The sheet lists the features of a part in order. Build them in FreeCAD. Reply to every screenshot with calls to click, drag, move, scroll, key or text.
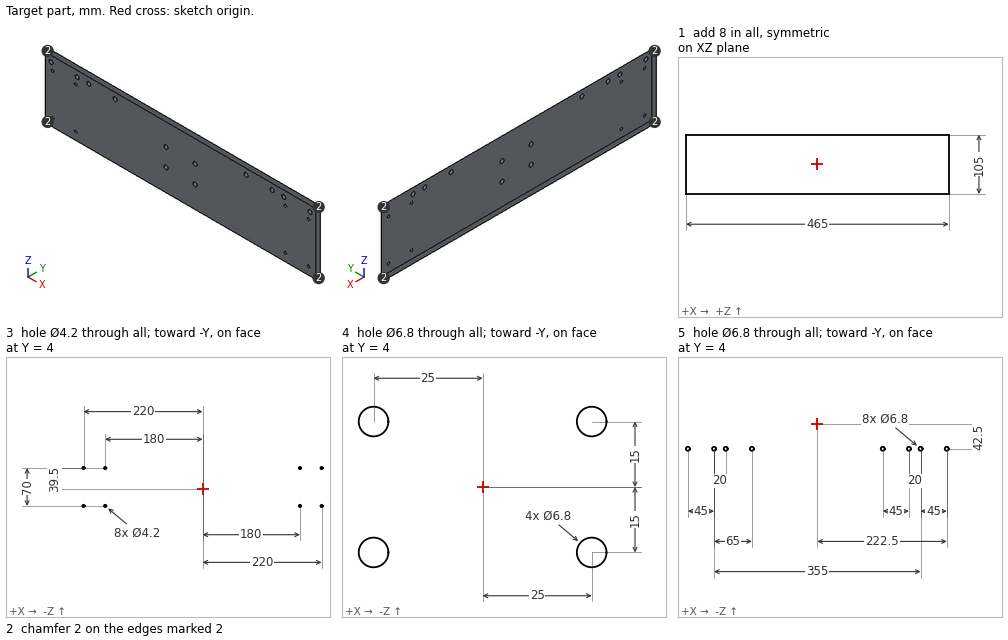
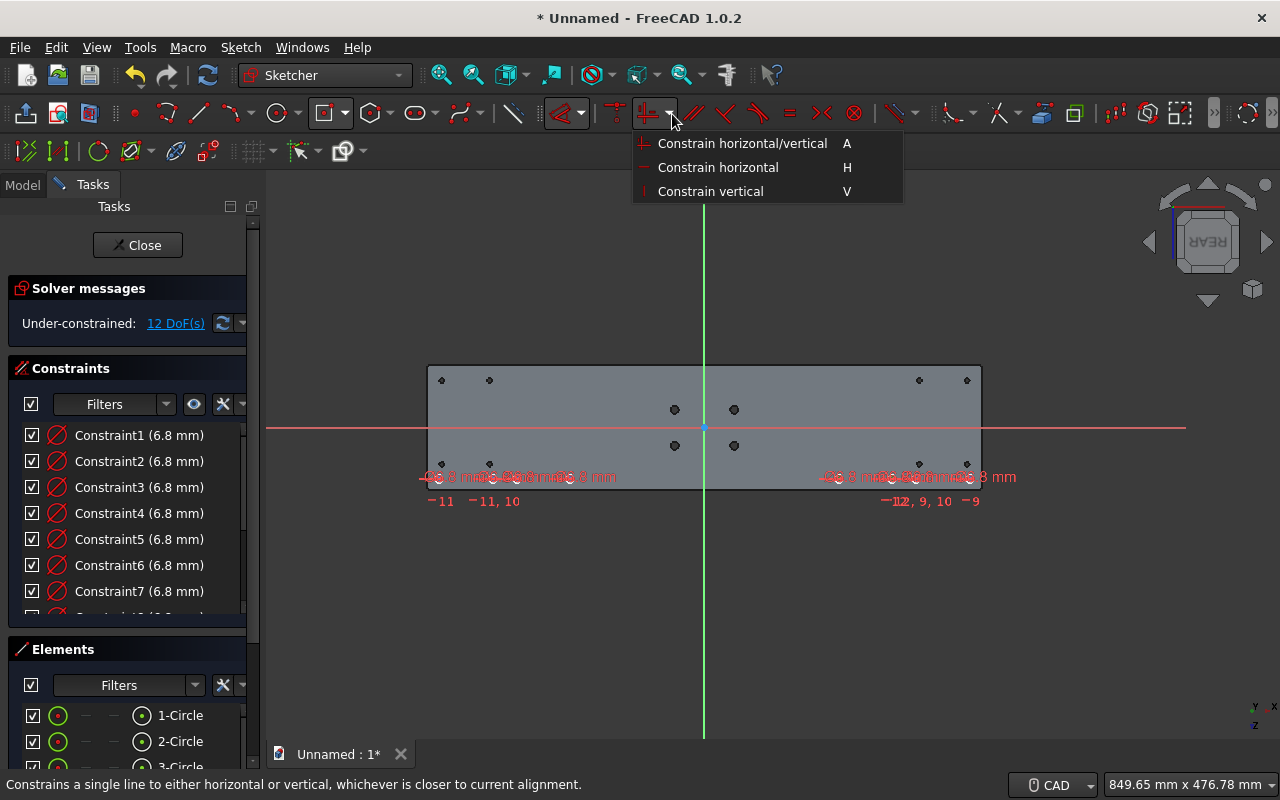
click(768, 167)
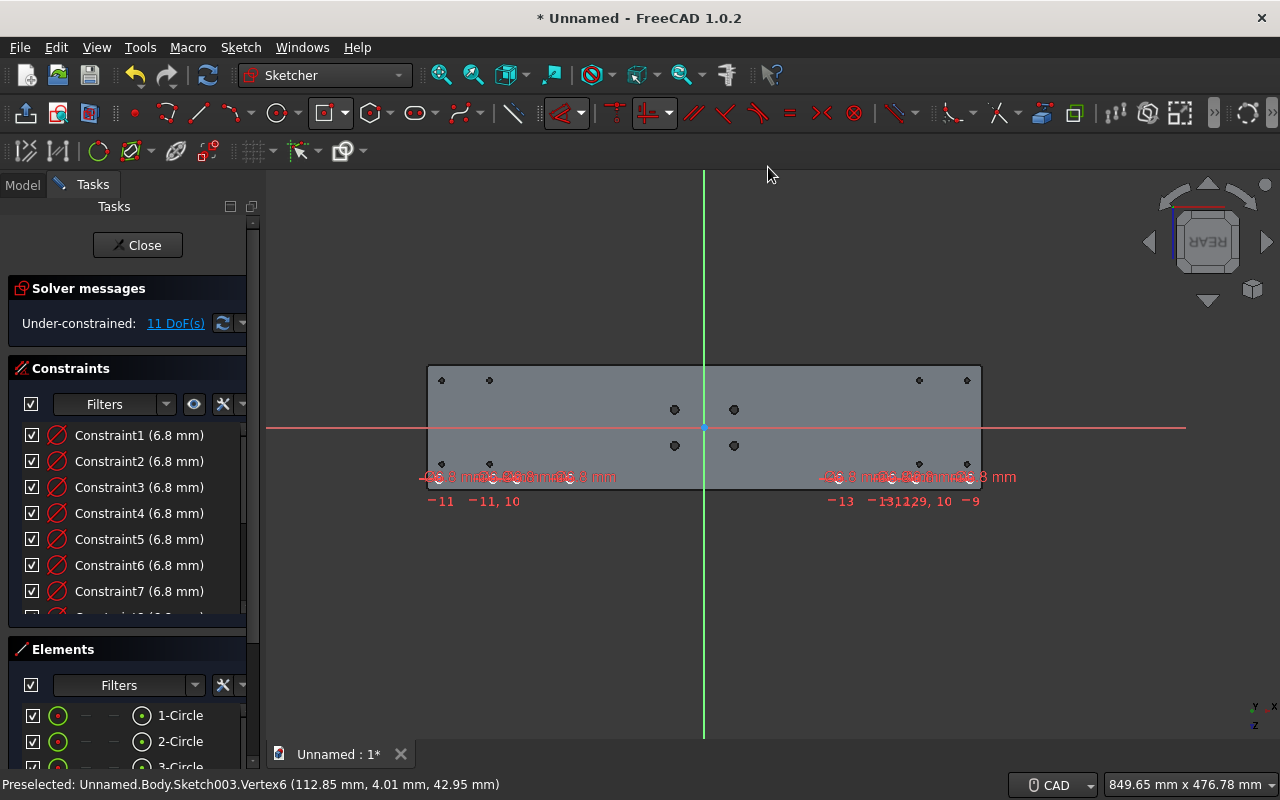
click(493, 479)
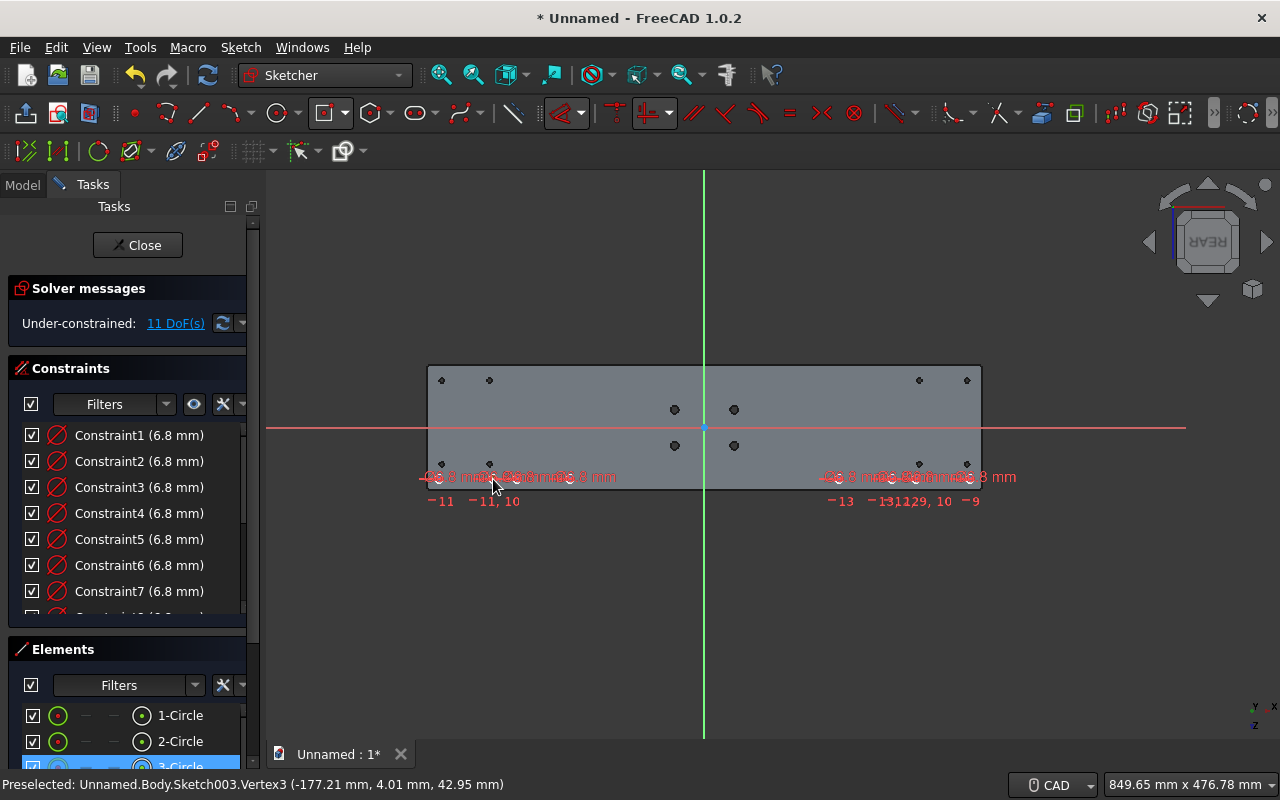
click(570, 479)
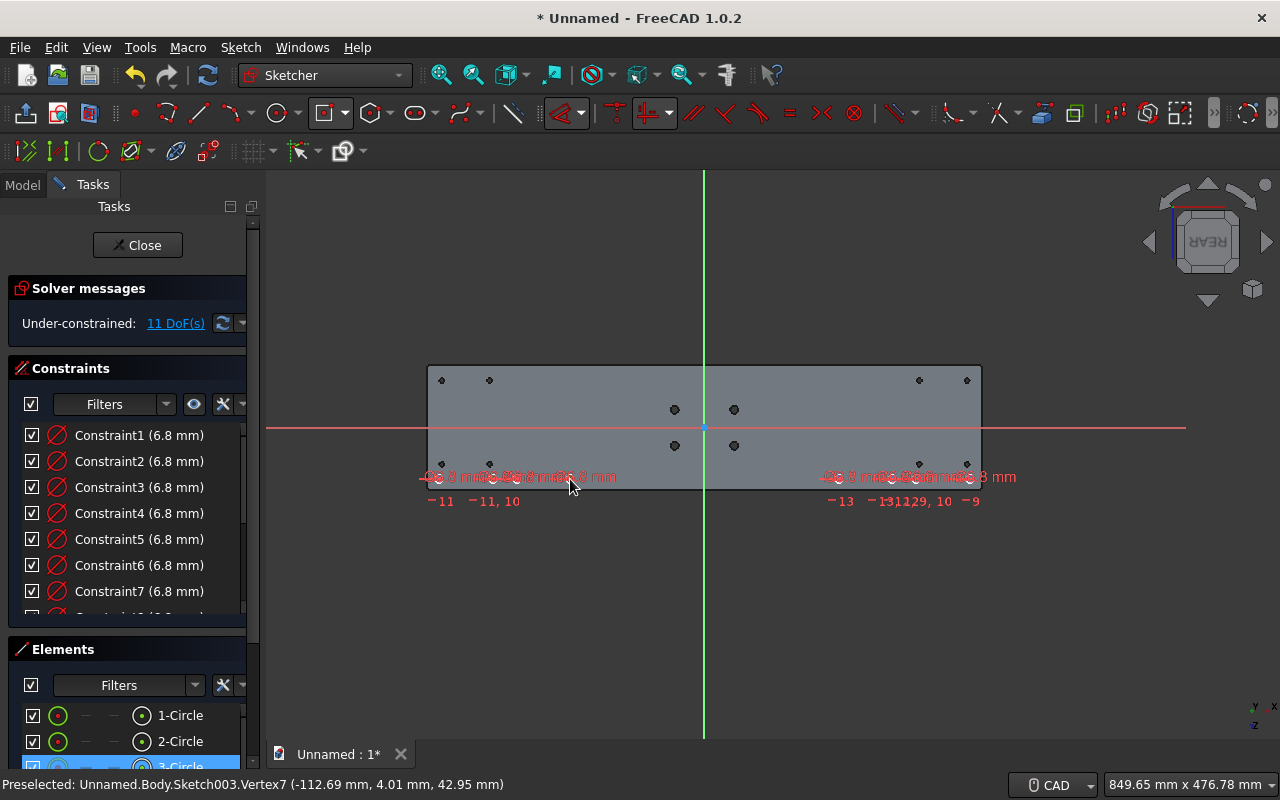
click(672, 114)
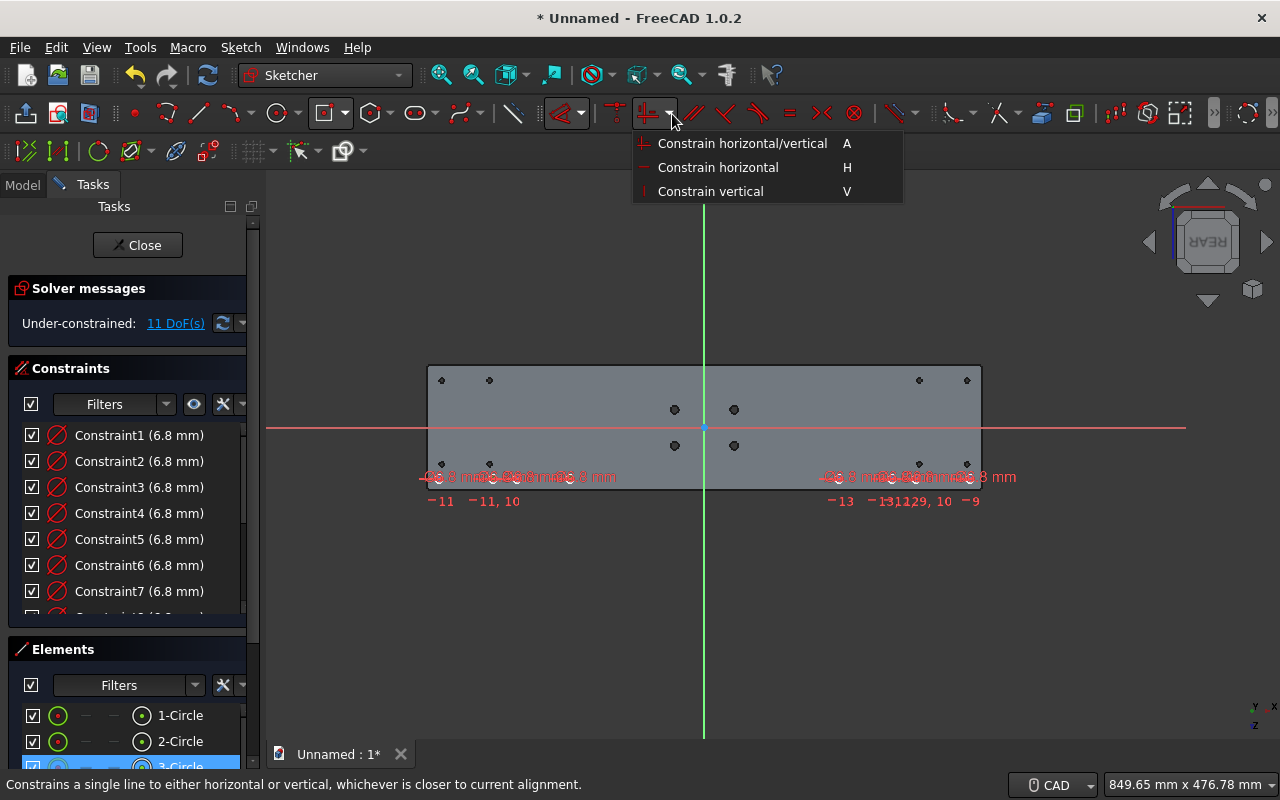
click(768, 167)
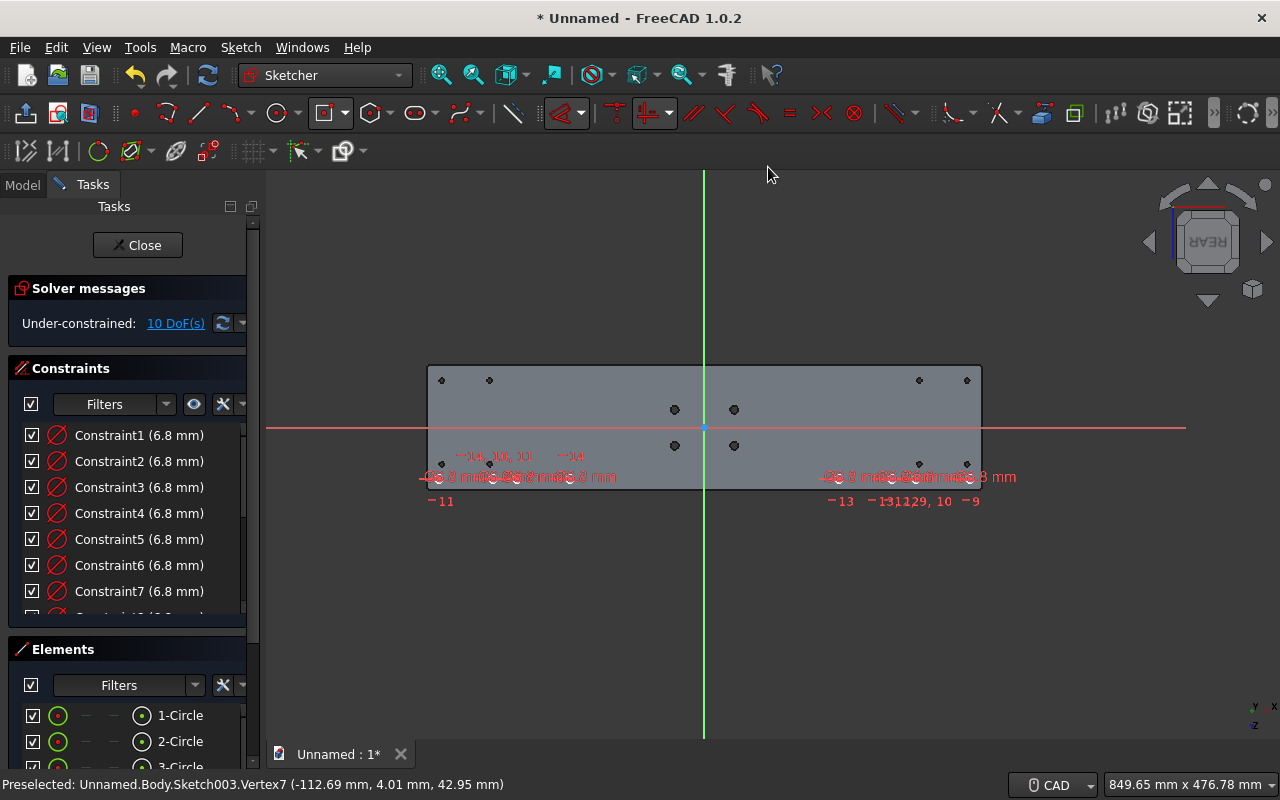
click(493, 479)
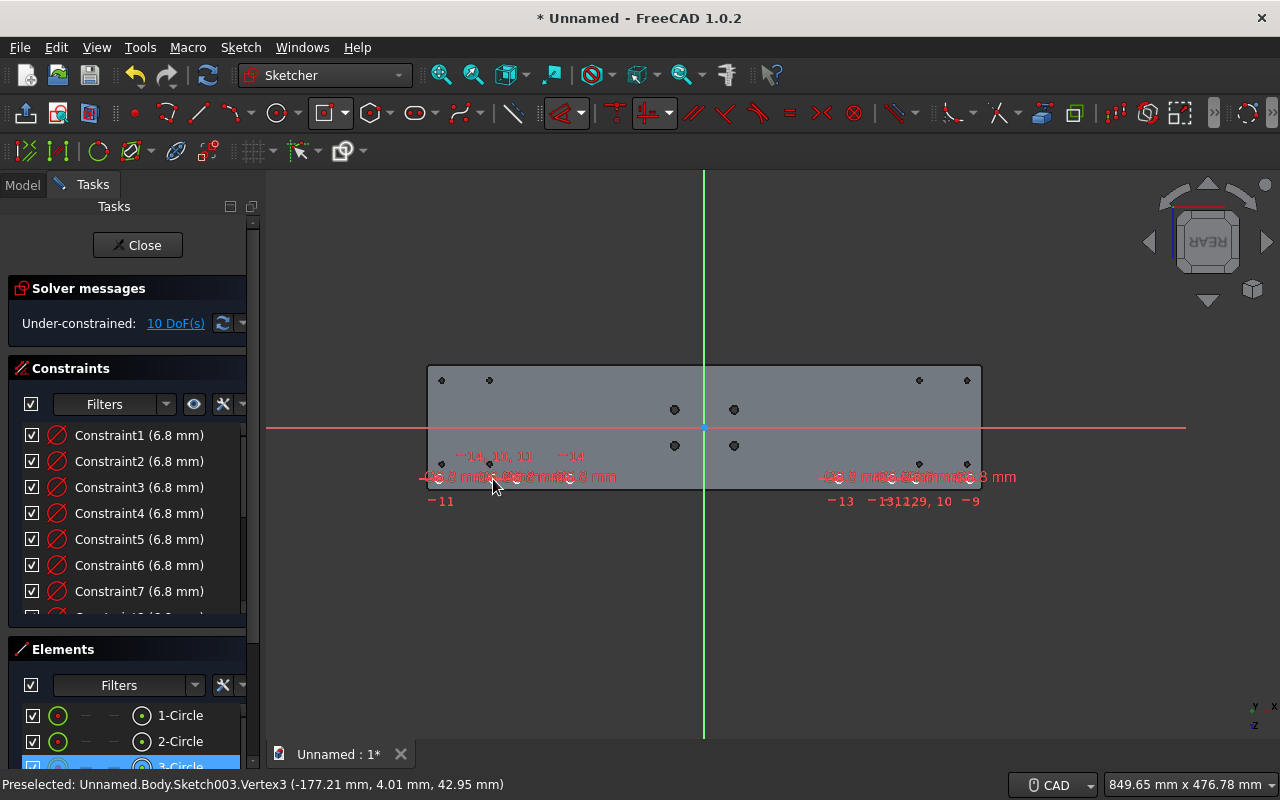
click(517, 479)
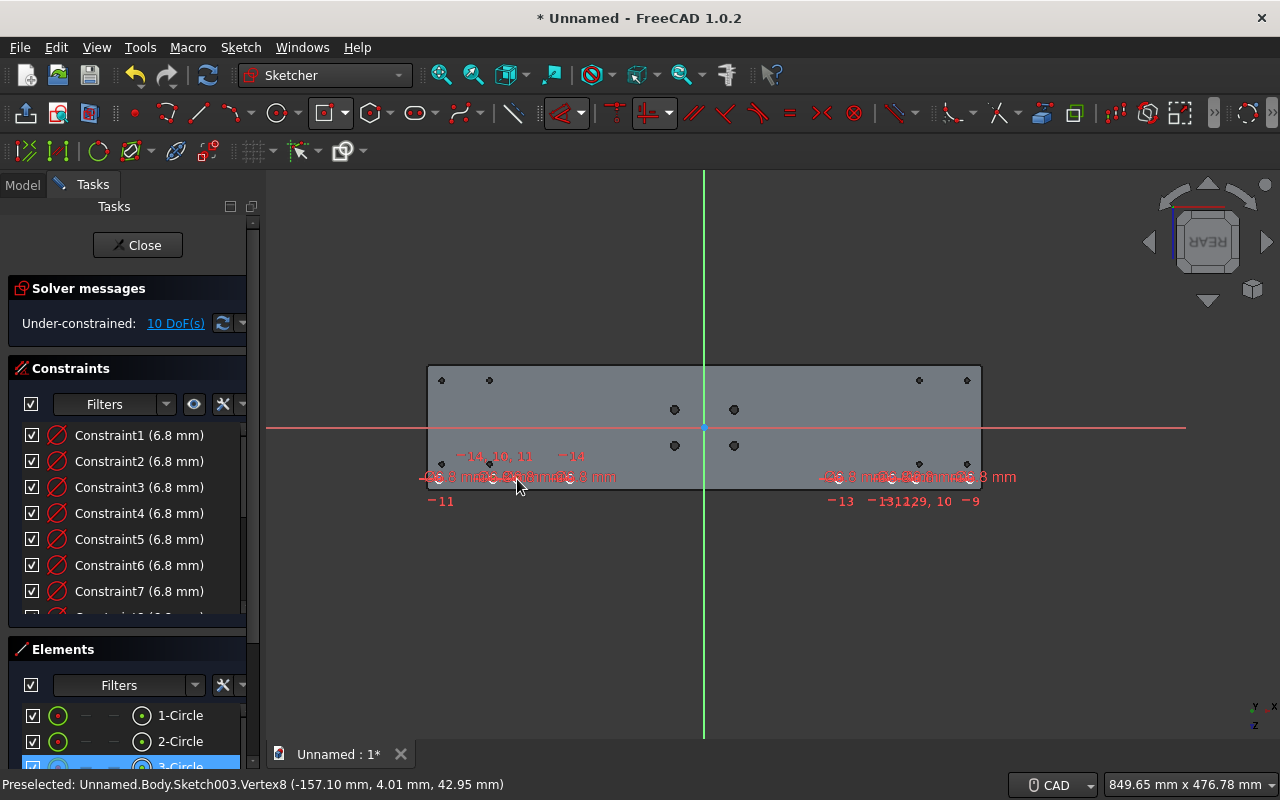
click(672, 114)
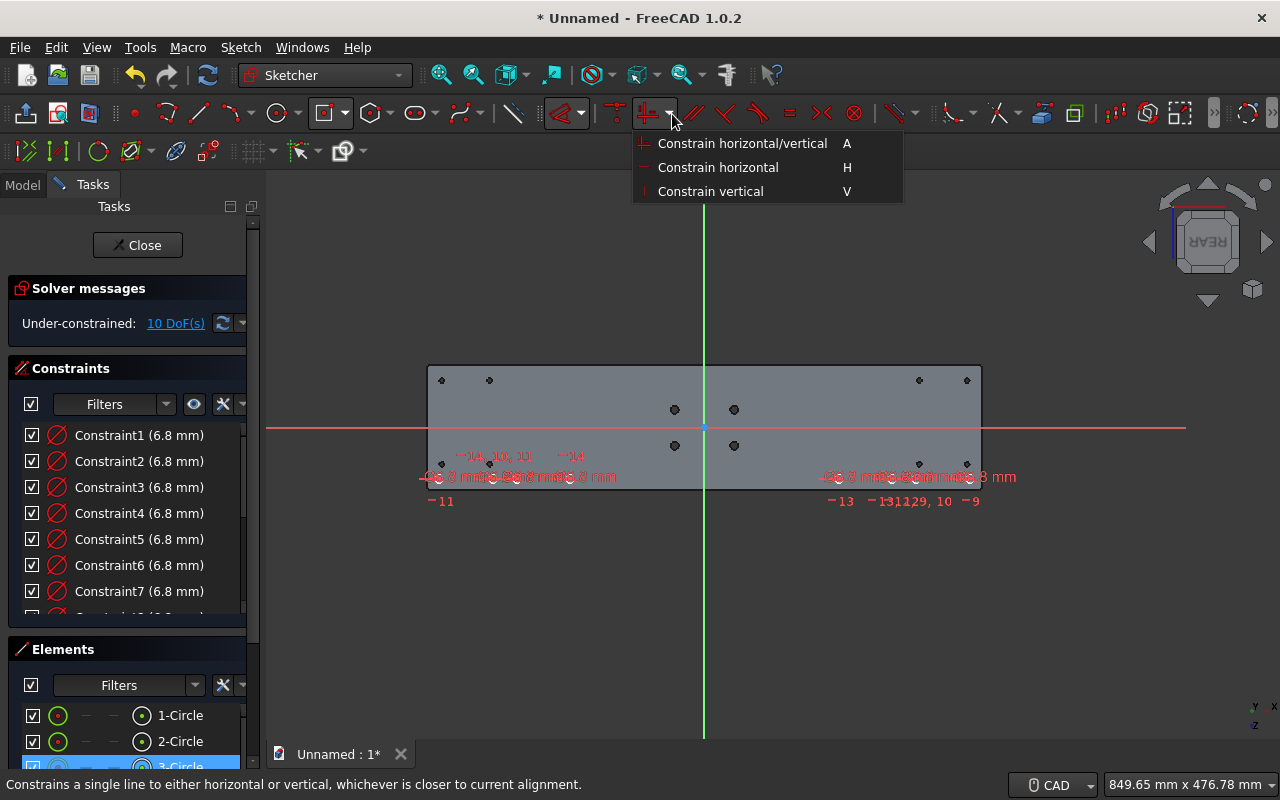
click(768, 167)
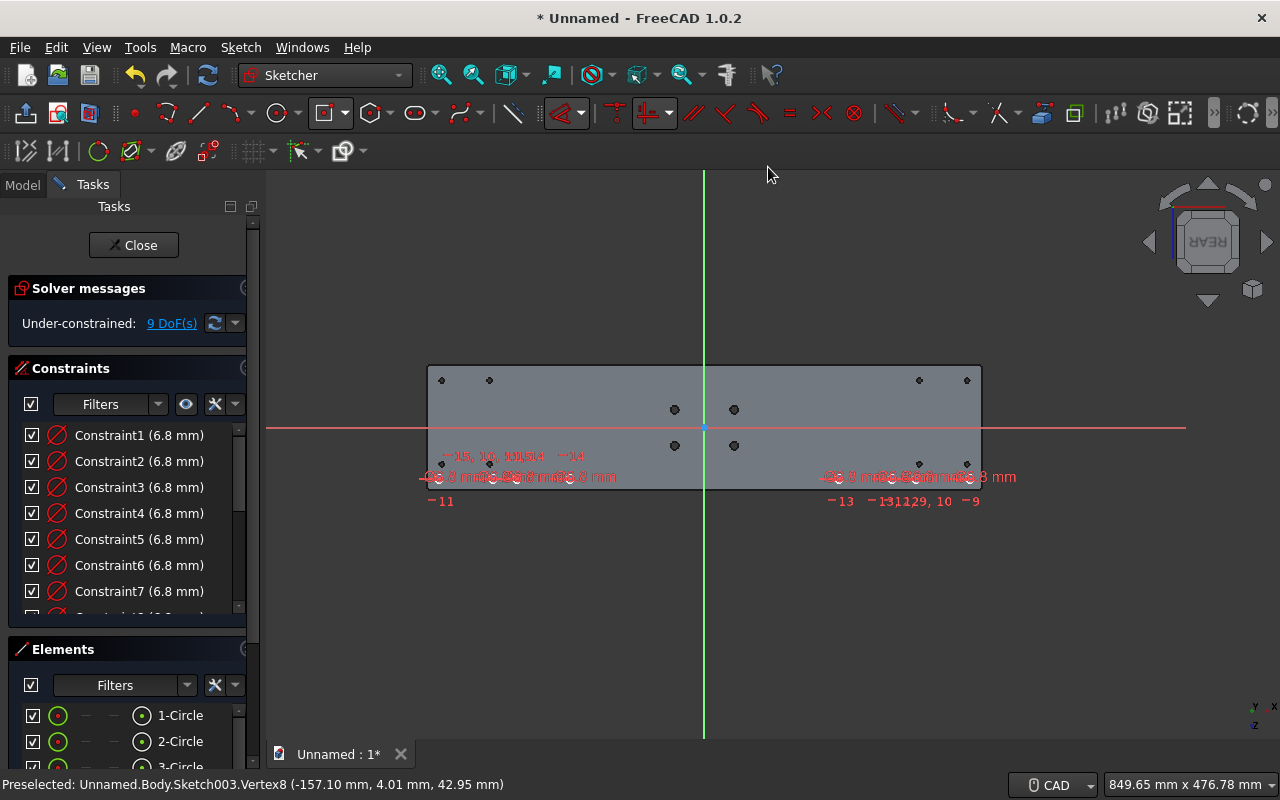
click(970, 479)